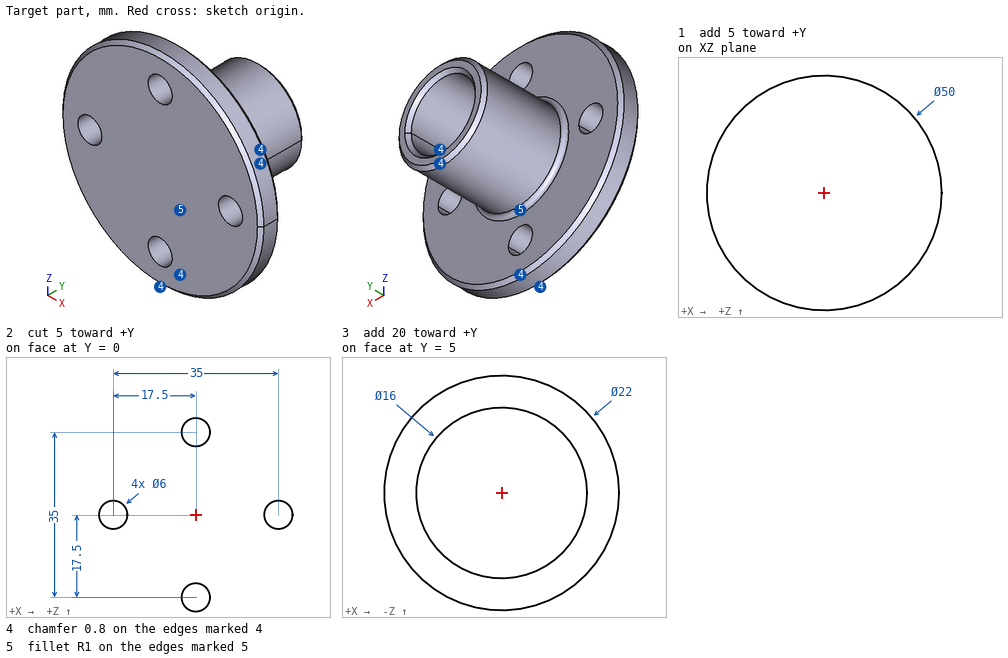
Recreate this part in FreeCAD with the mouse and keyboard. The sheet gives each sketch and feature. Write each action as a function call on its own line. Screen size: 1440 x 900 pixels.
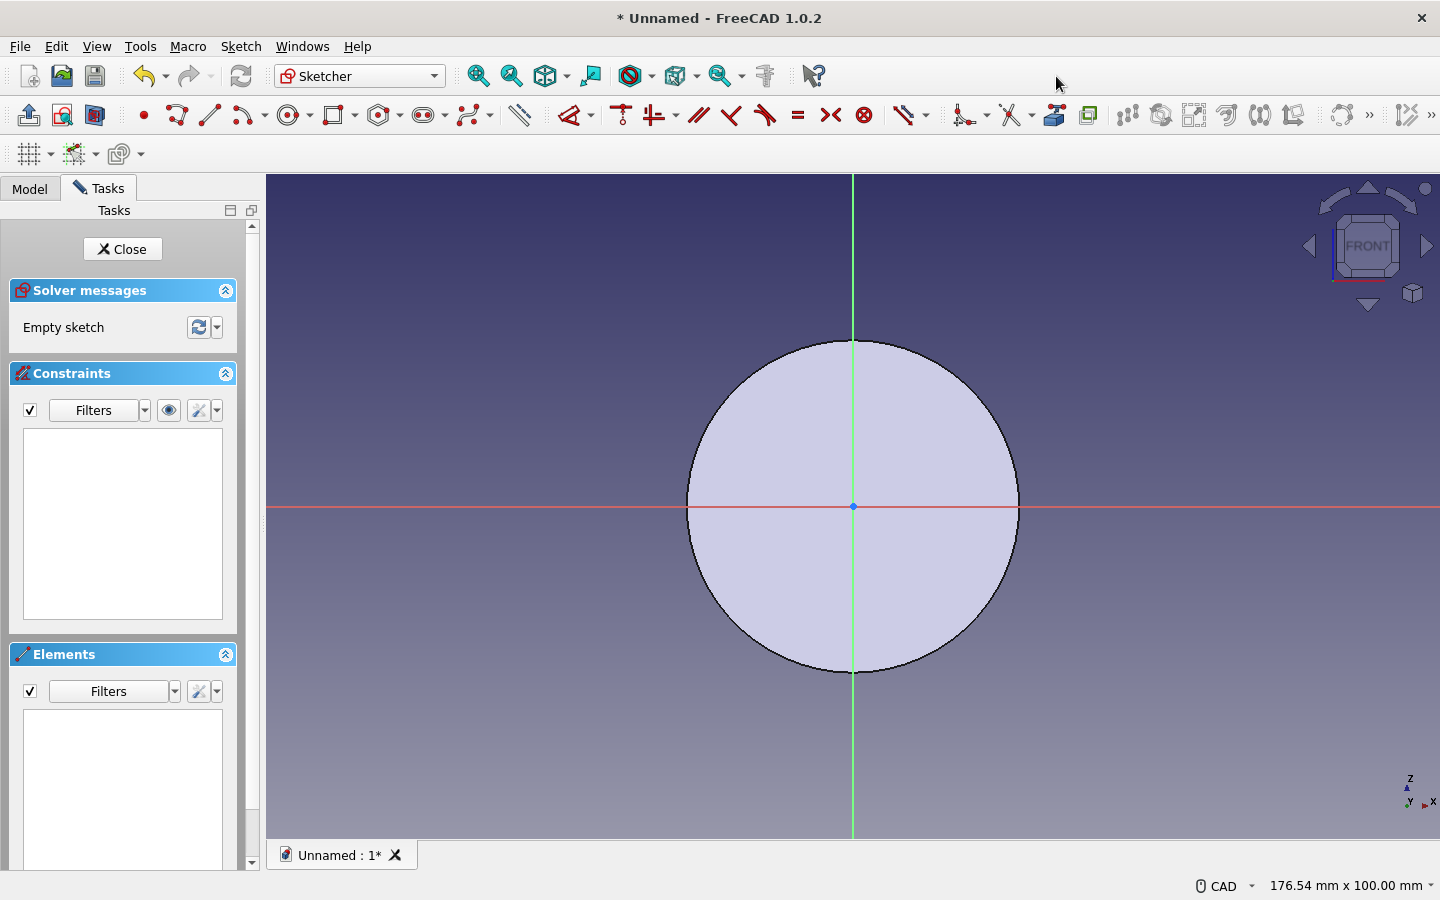
scroll(992, 506, up, 2)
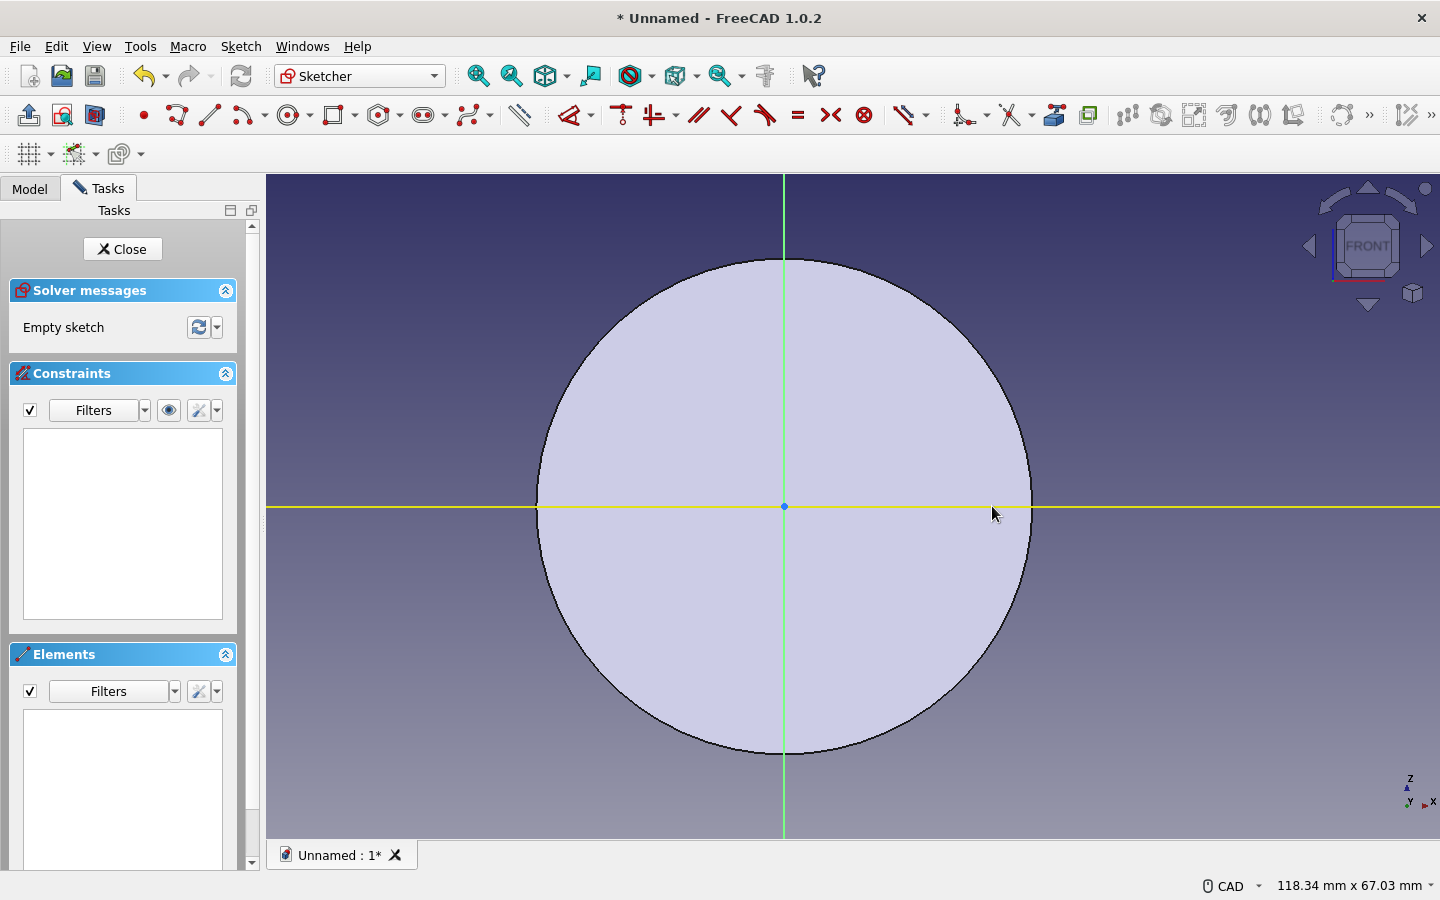
click(288, 116)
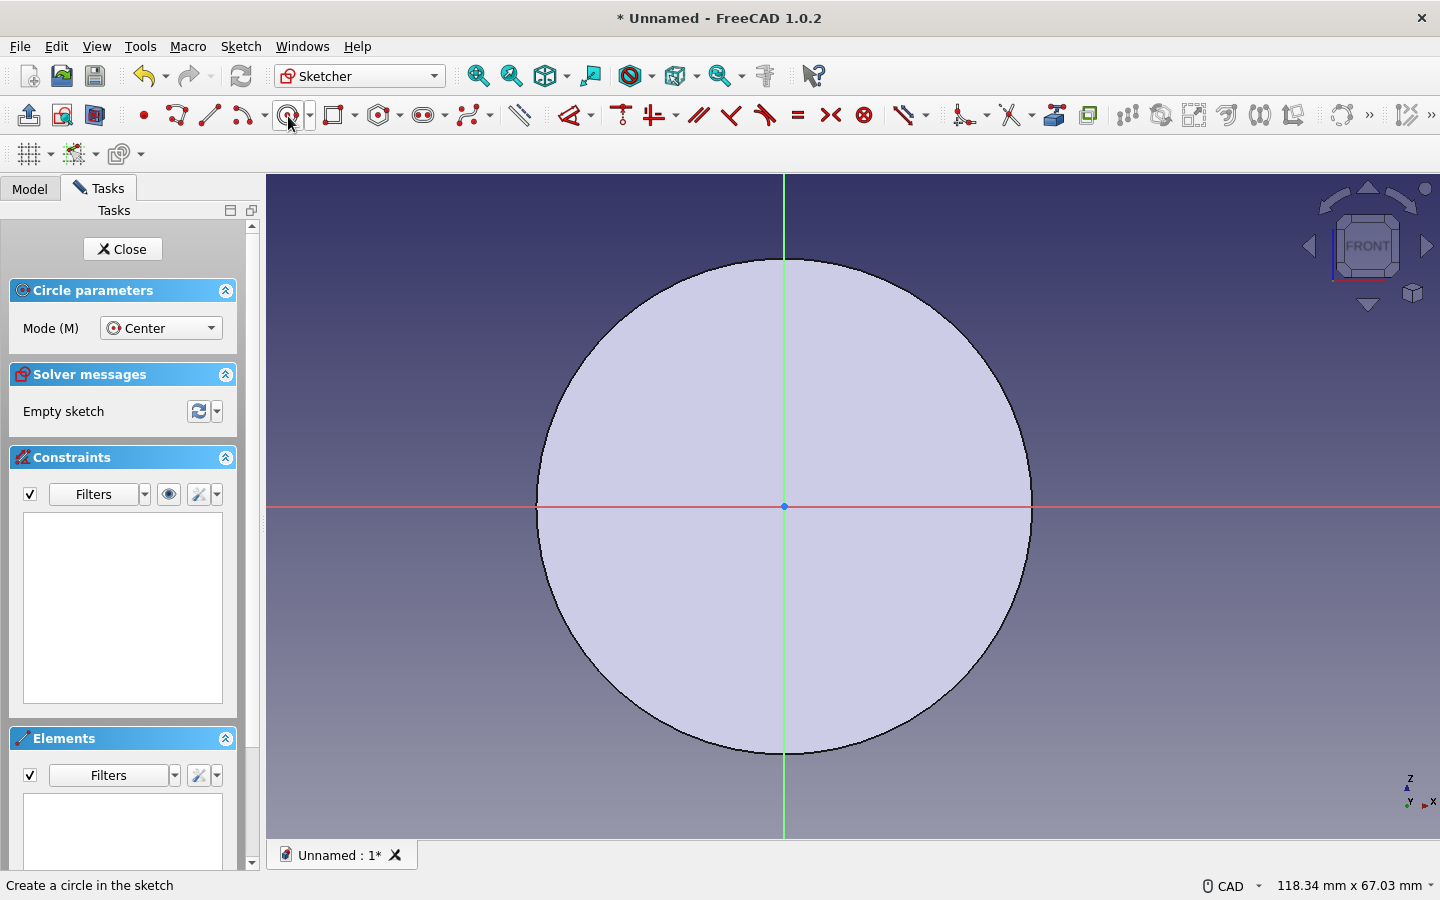
click(611, 506)
click(632, 485)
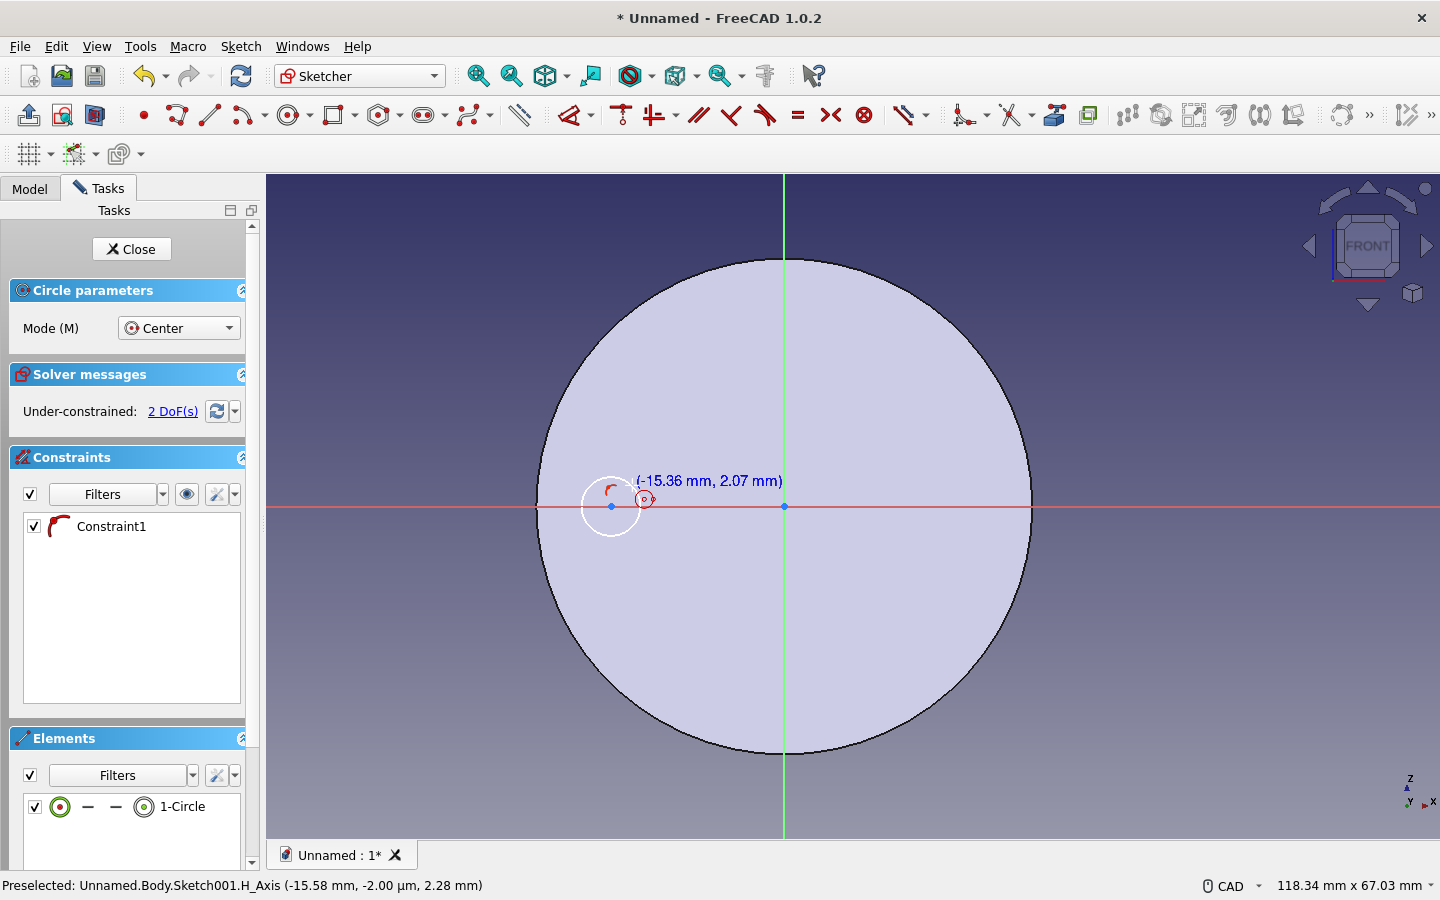
click(784, 680)
click(805, 659)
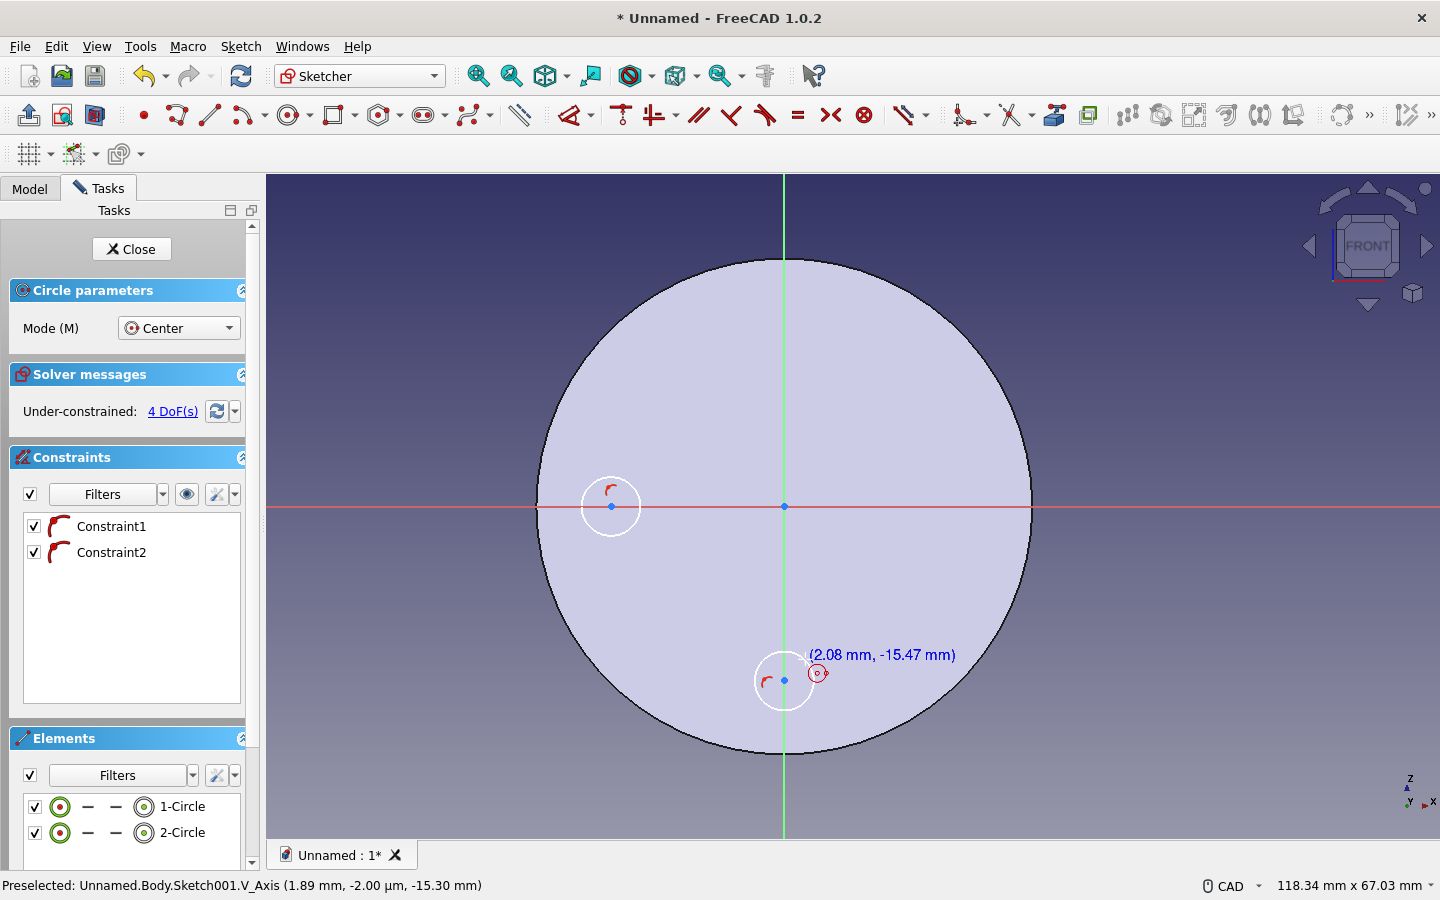
click(958, 506)
click(979, 485)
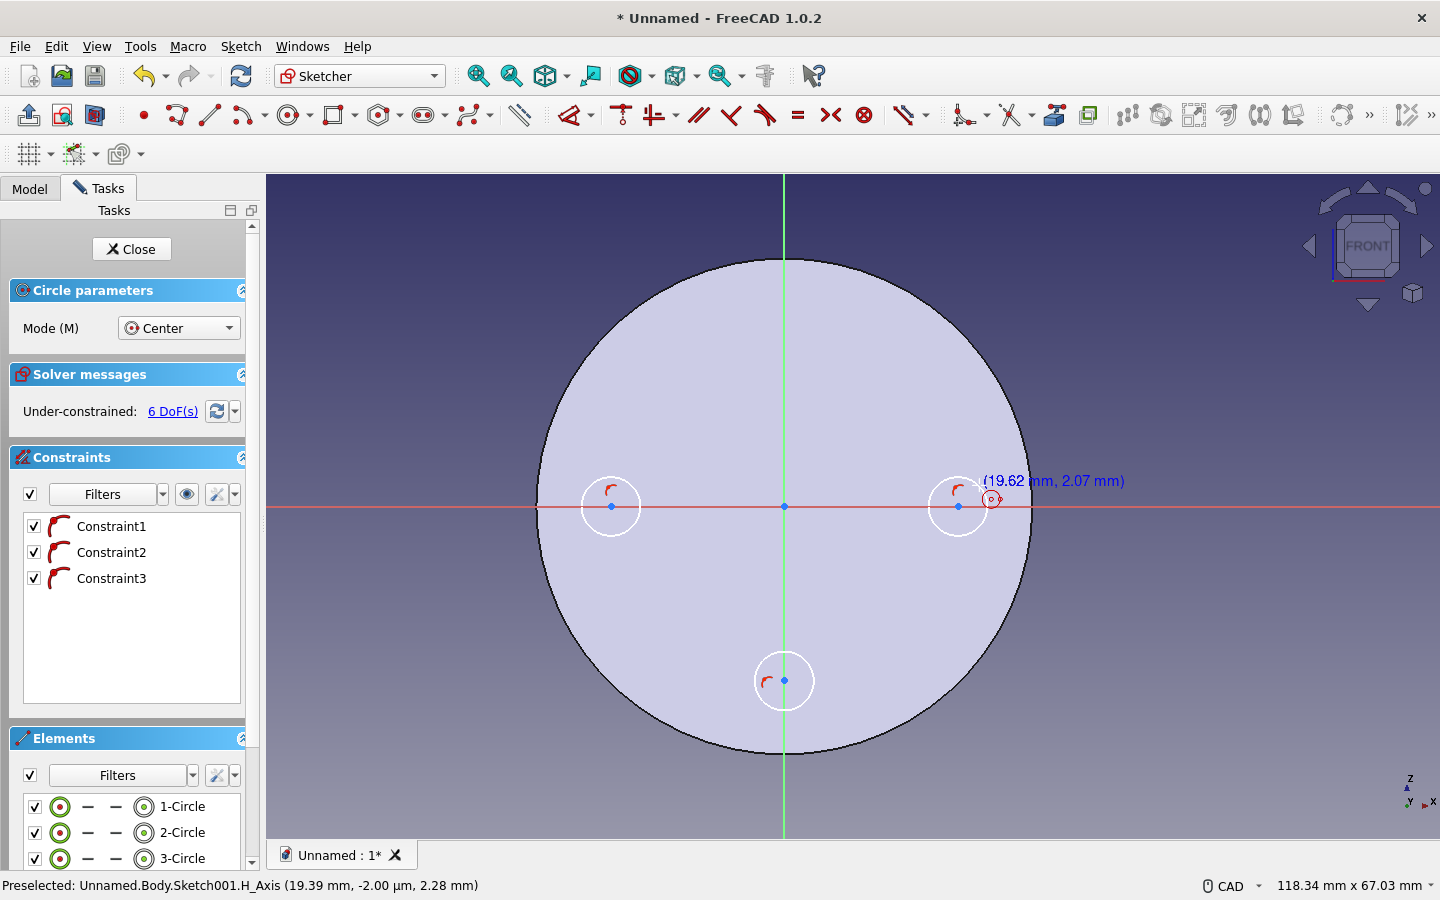
click(784, 333)
click(805, 312)
key(Escape)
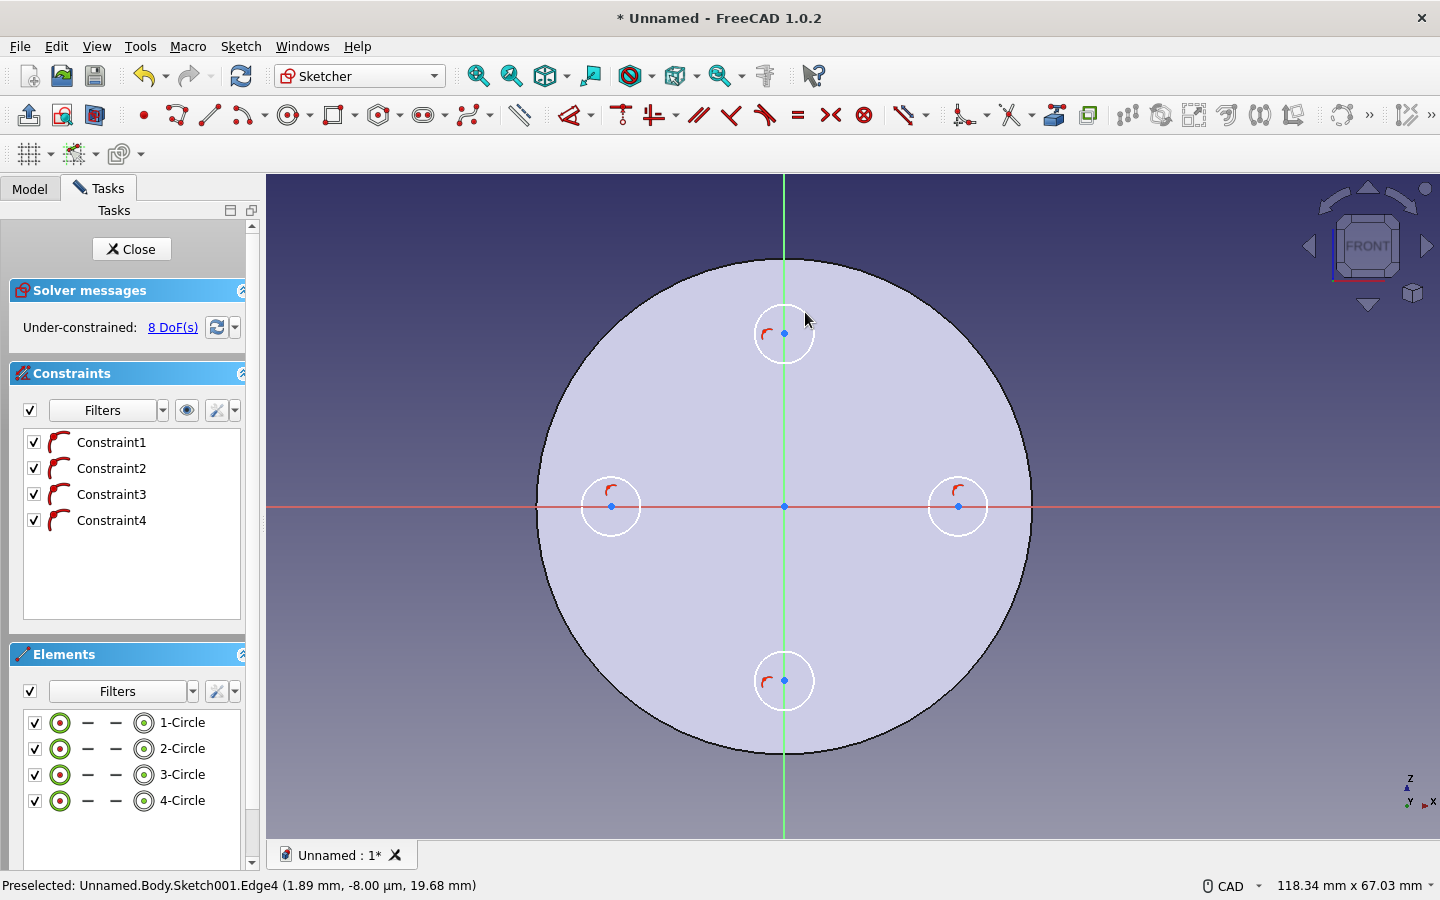
click(632, 486)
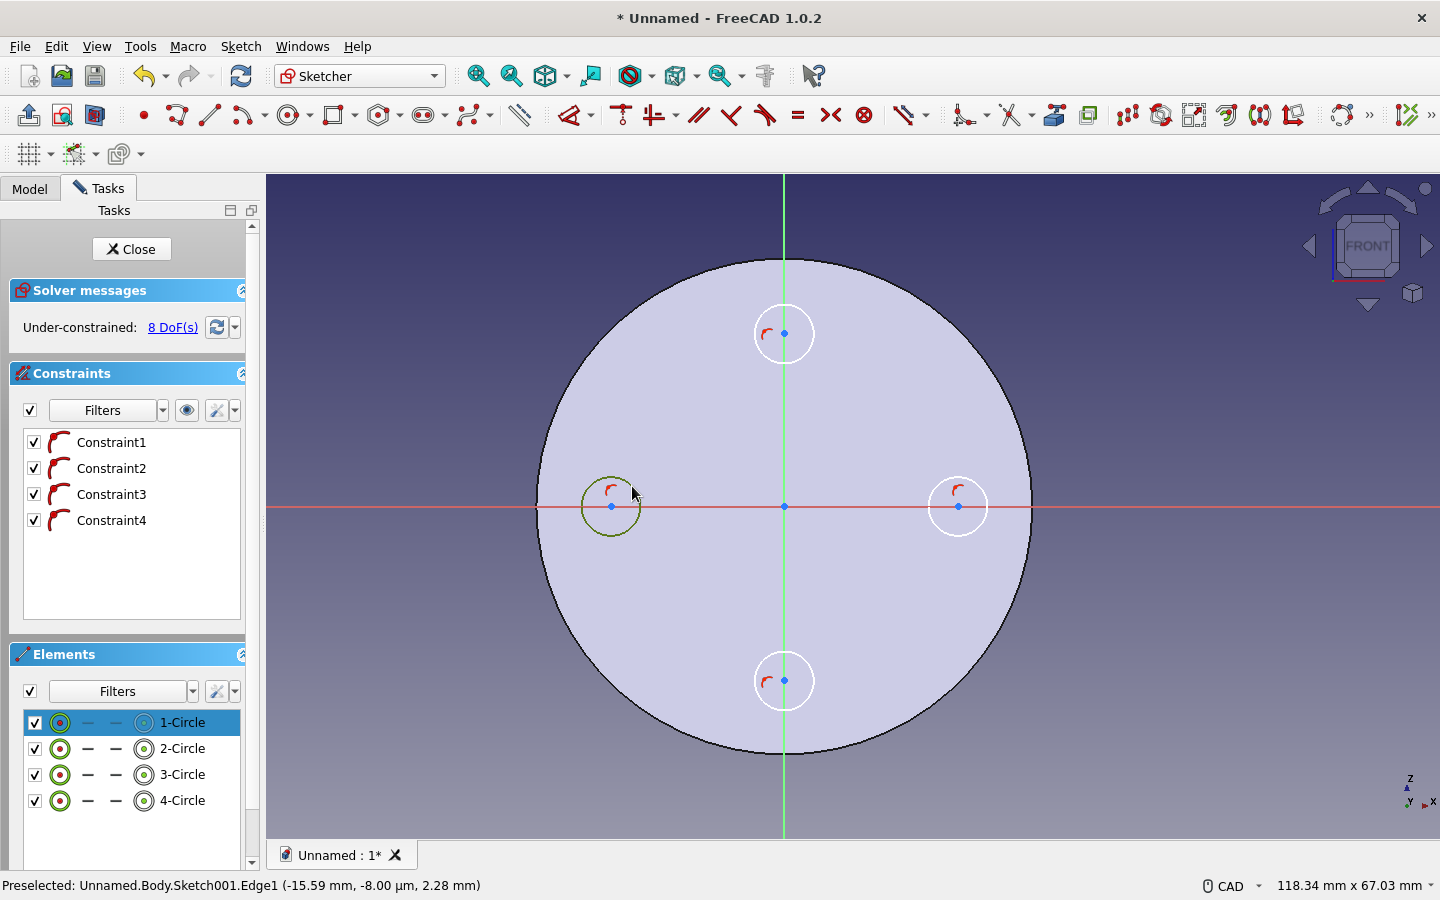
click(805, 660)